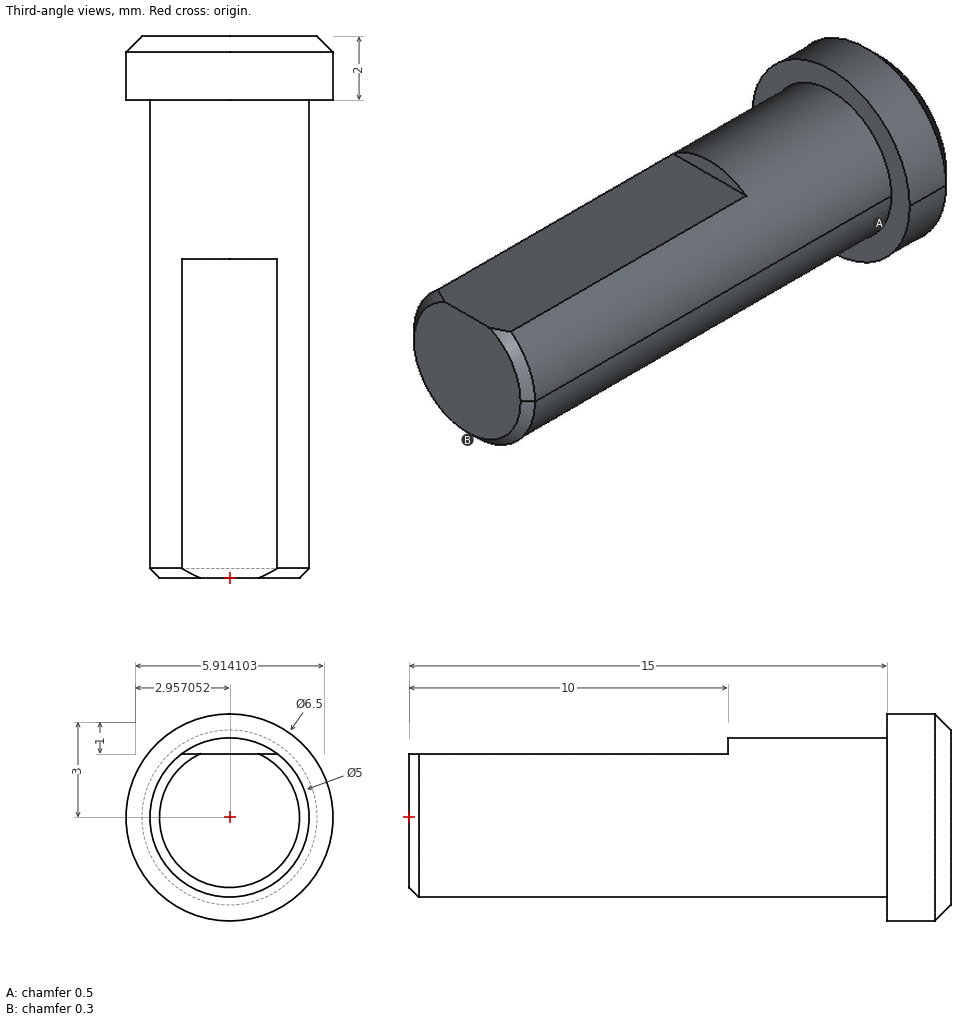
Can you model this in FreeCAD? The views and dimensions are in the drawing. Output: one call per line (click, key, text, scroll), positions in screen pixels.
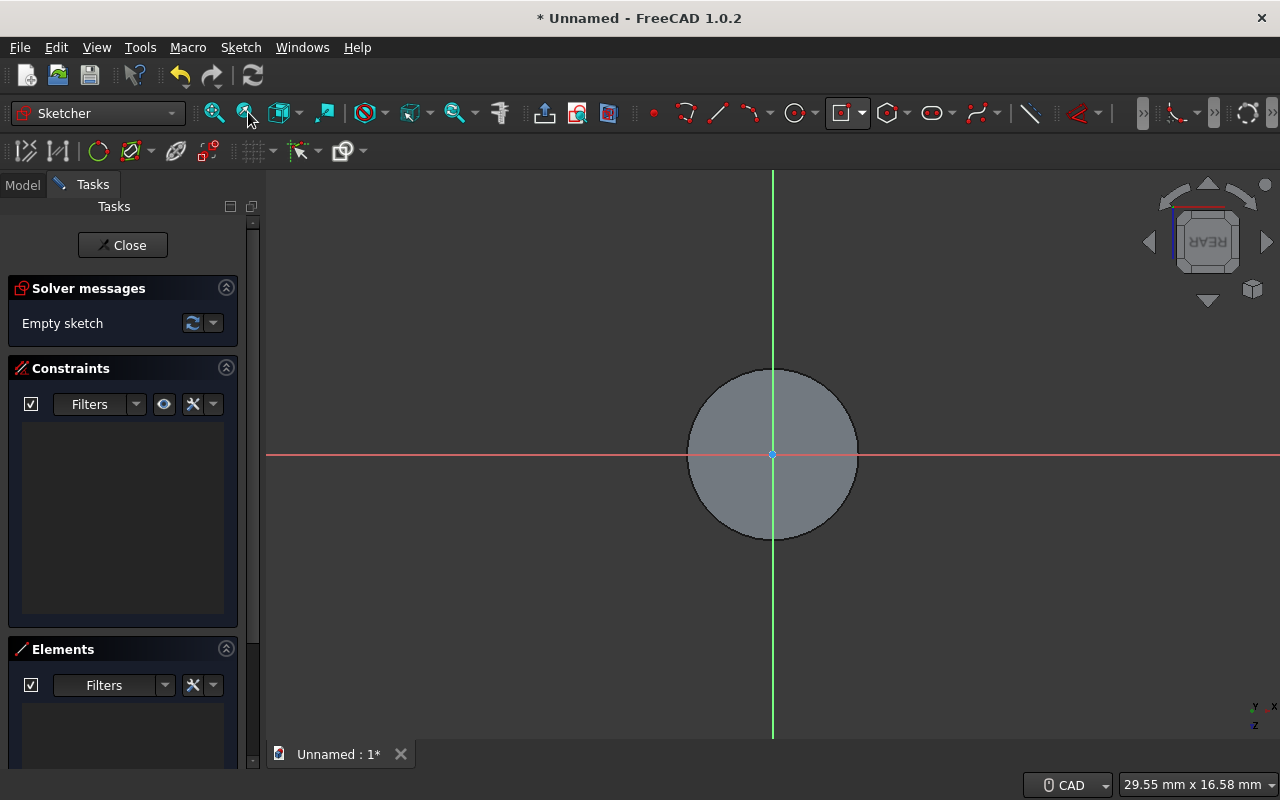
scroll(912, 454, up, 2)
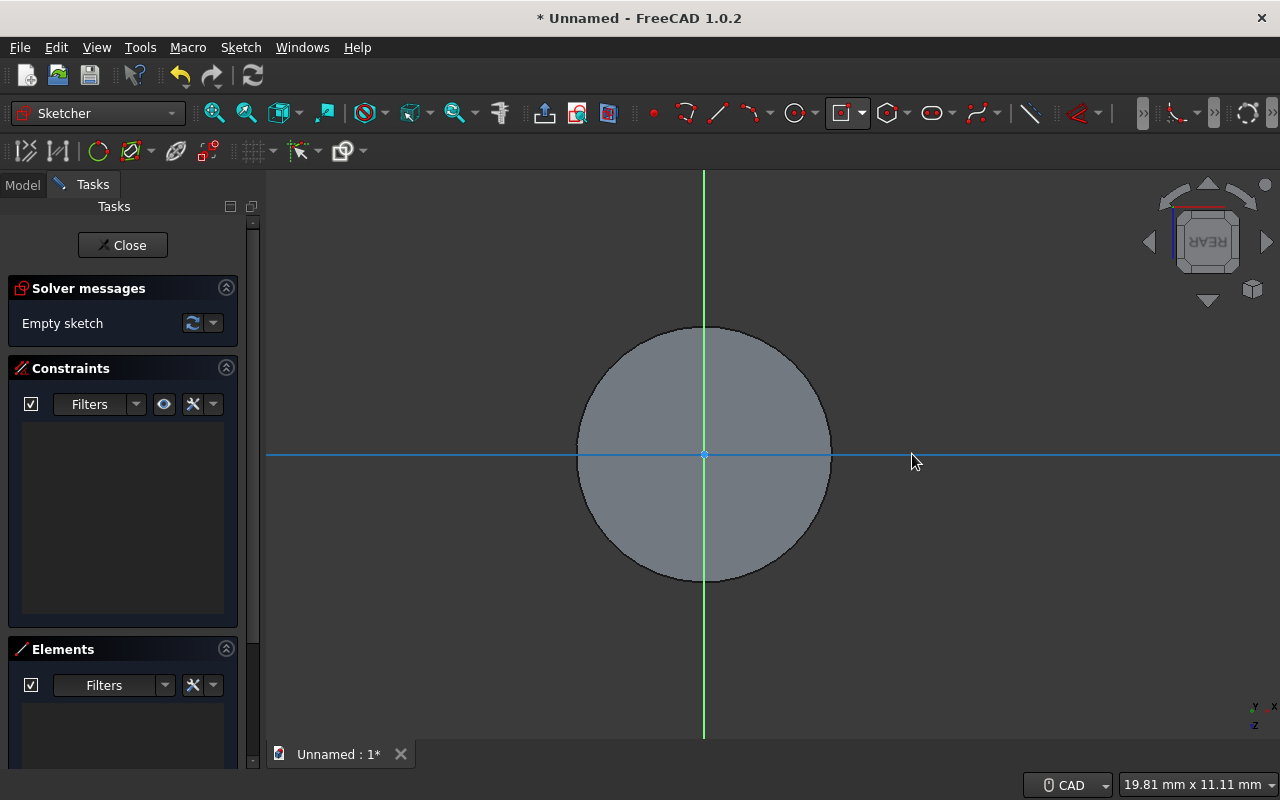
click(796, 114)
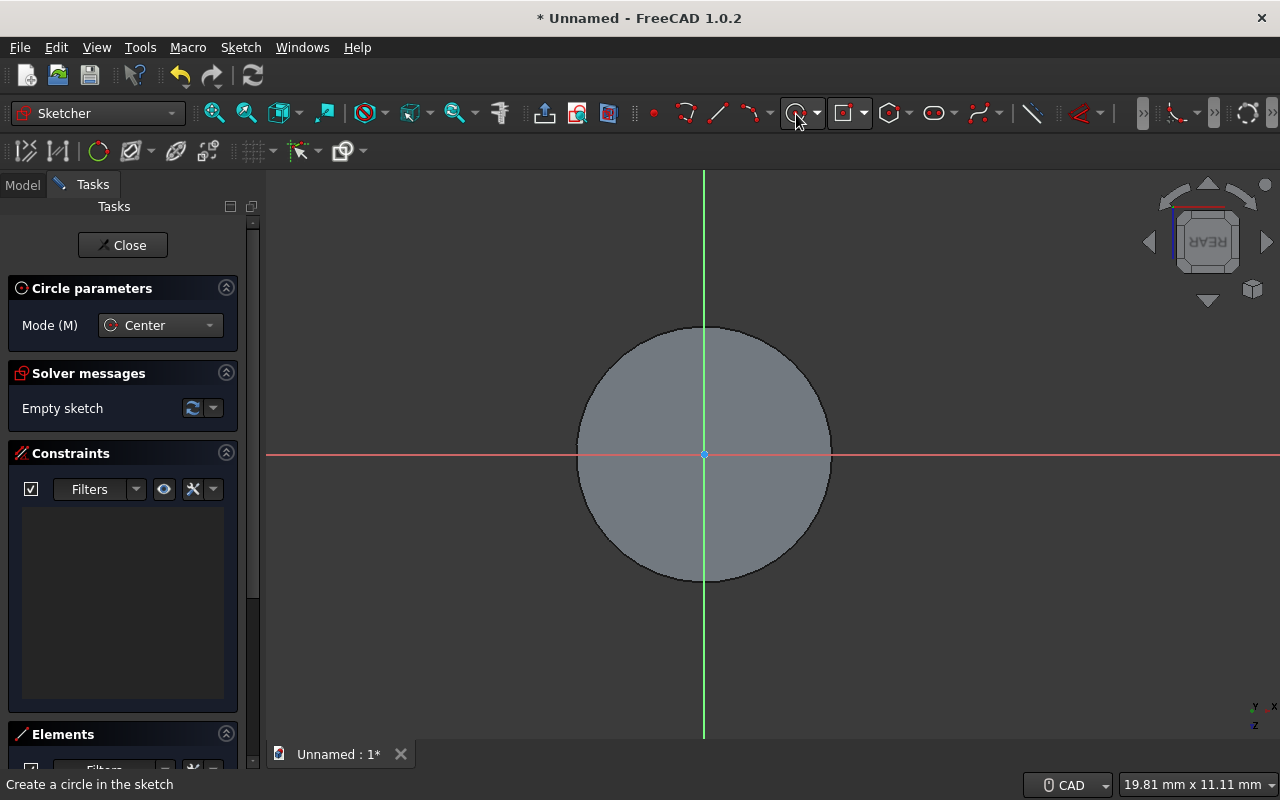
click(704, 454)
click(822, 337)
key(Escape)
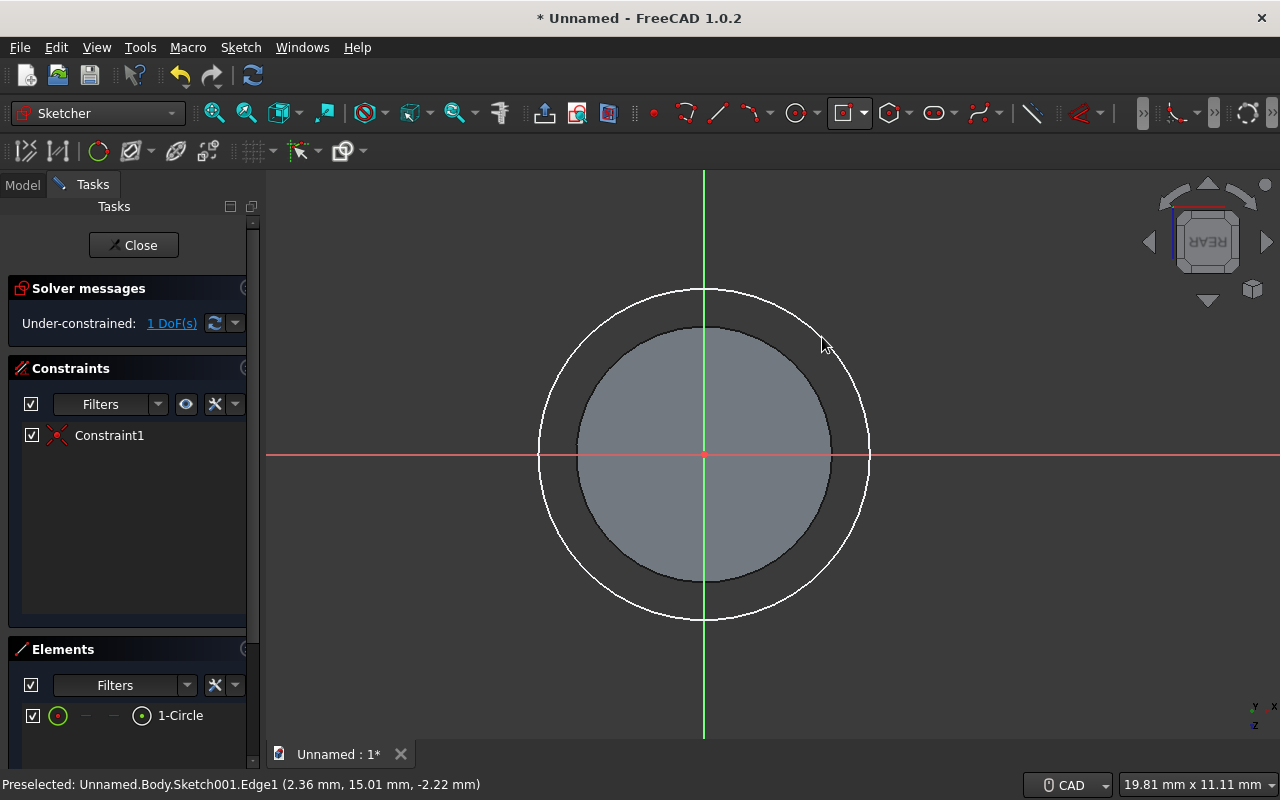
click(1080, 114)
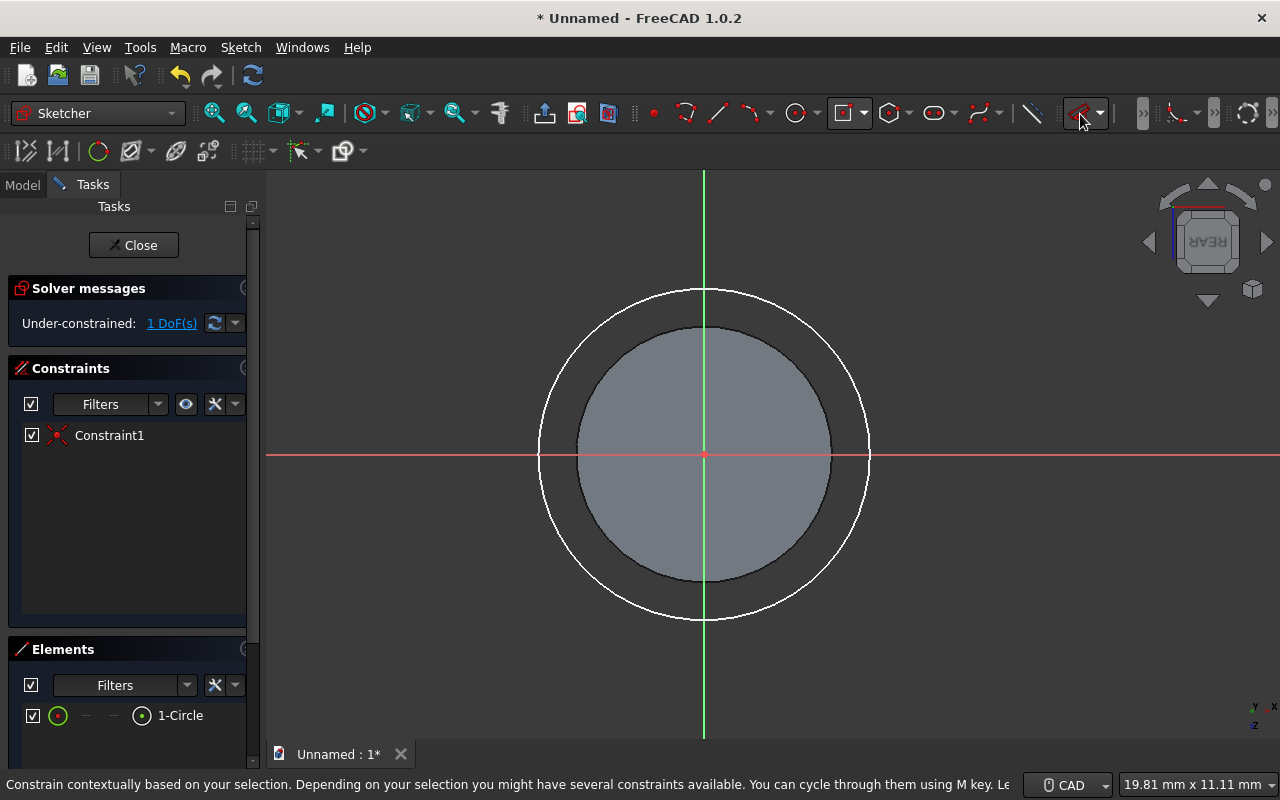
click(821, 337)
click(844, 314)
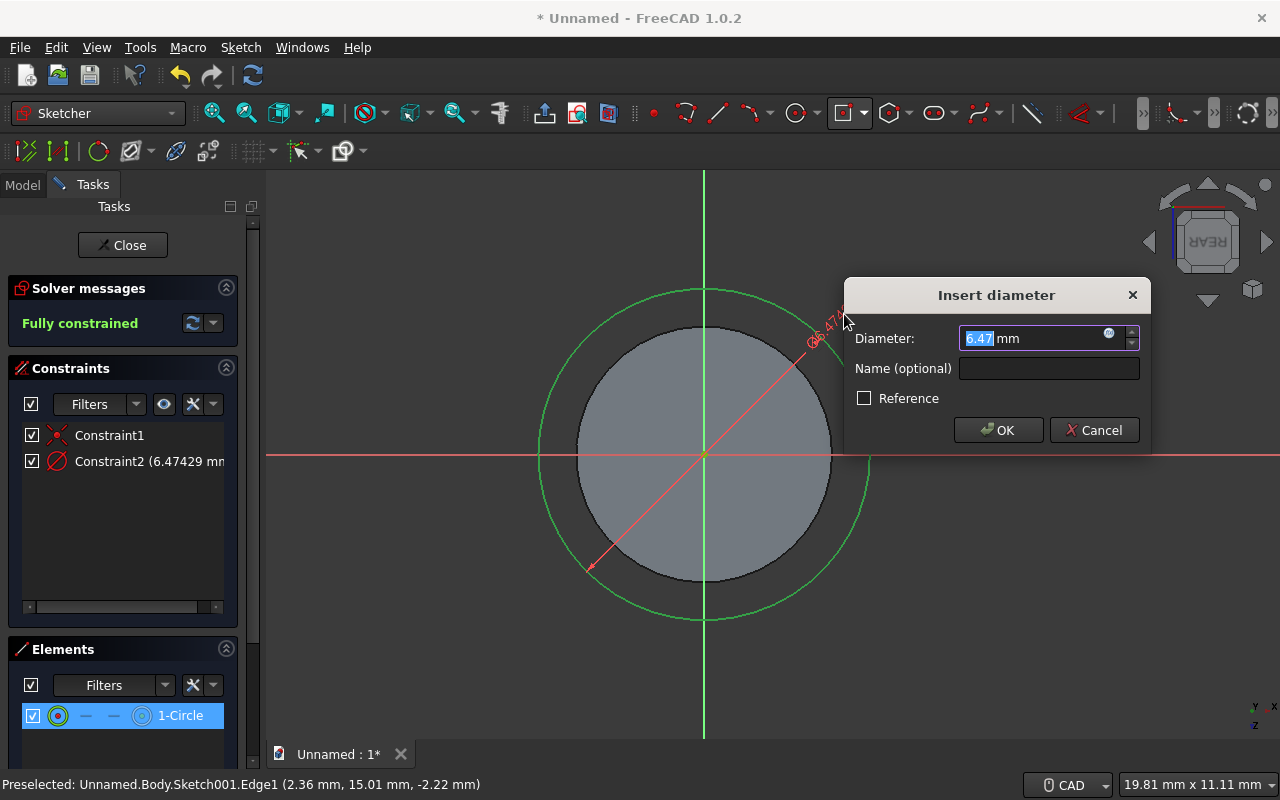
text(6.5)
key(Return)
key(Escape)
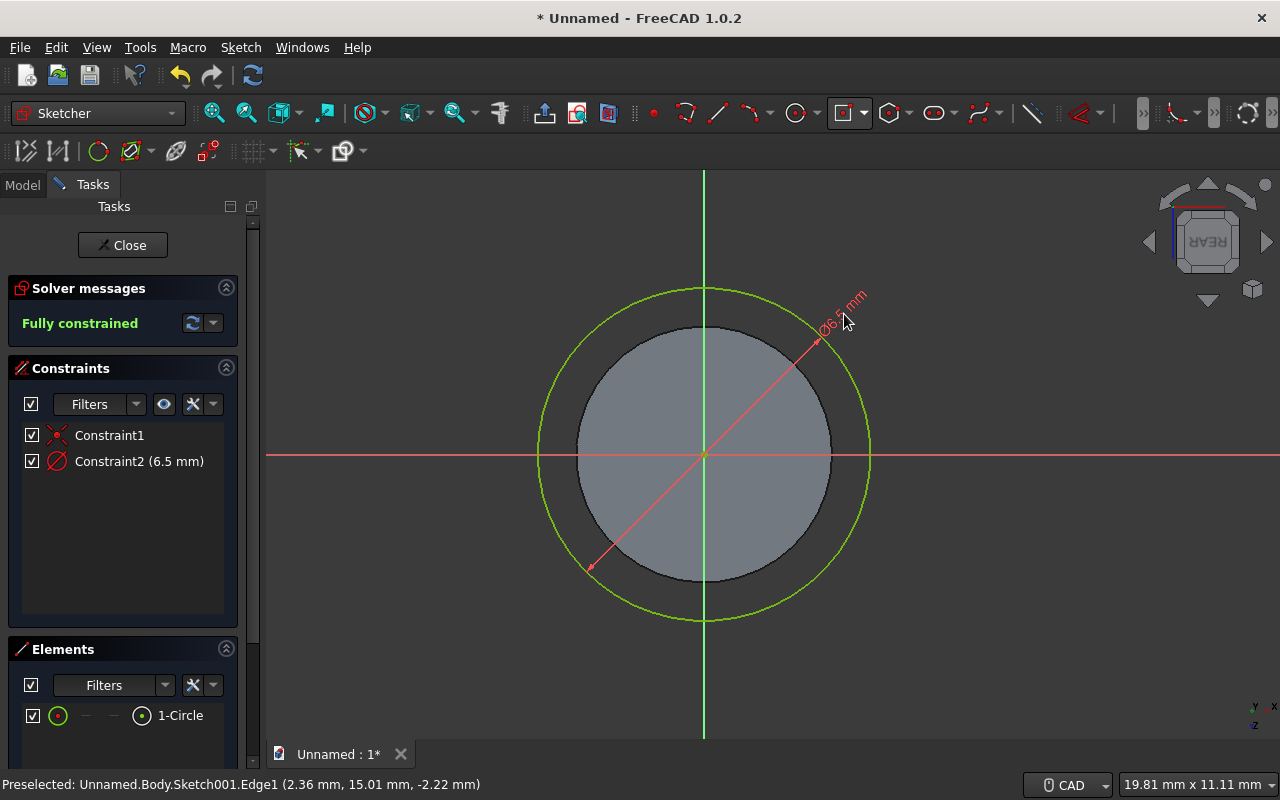
click(123, 245)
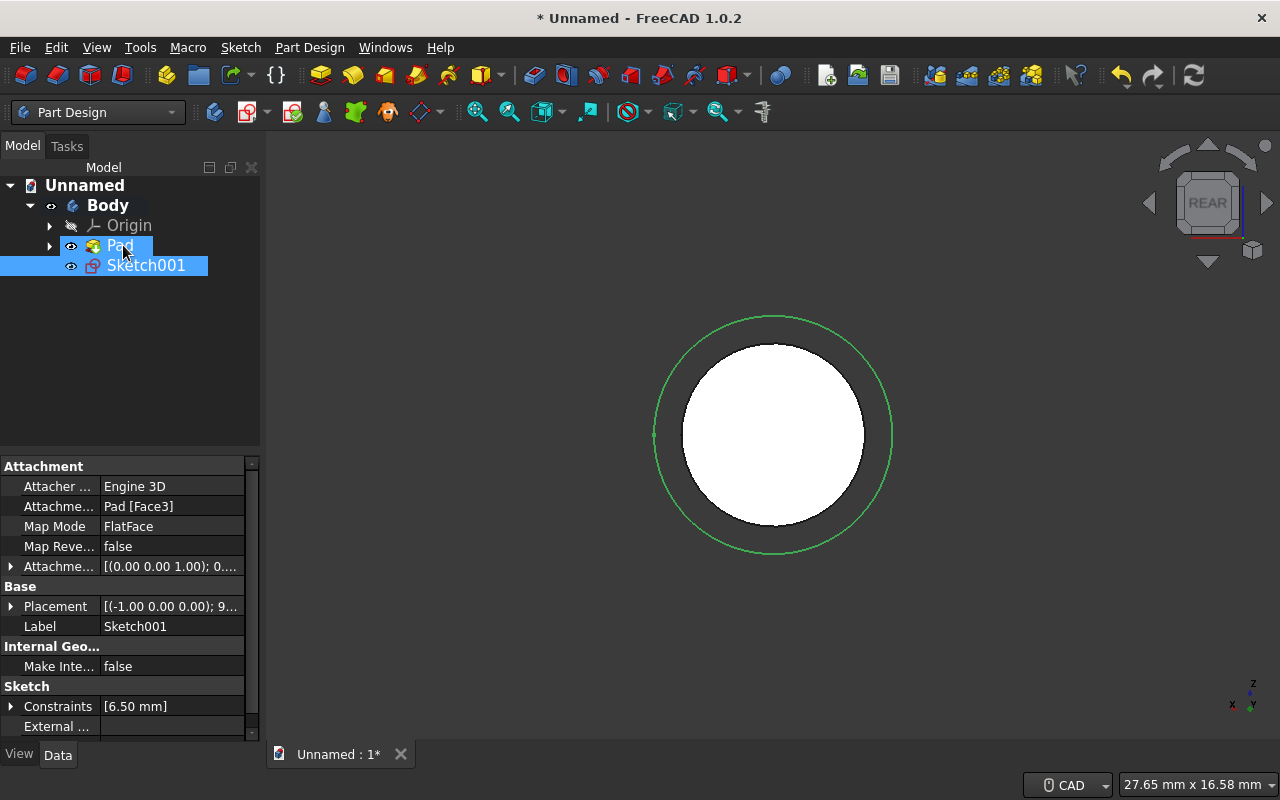
click(322, 76)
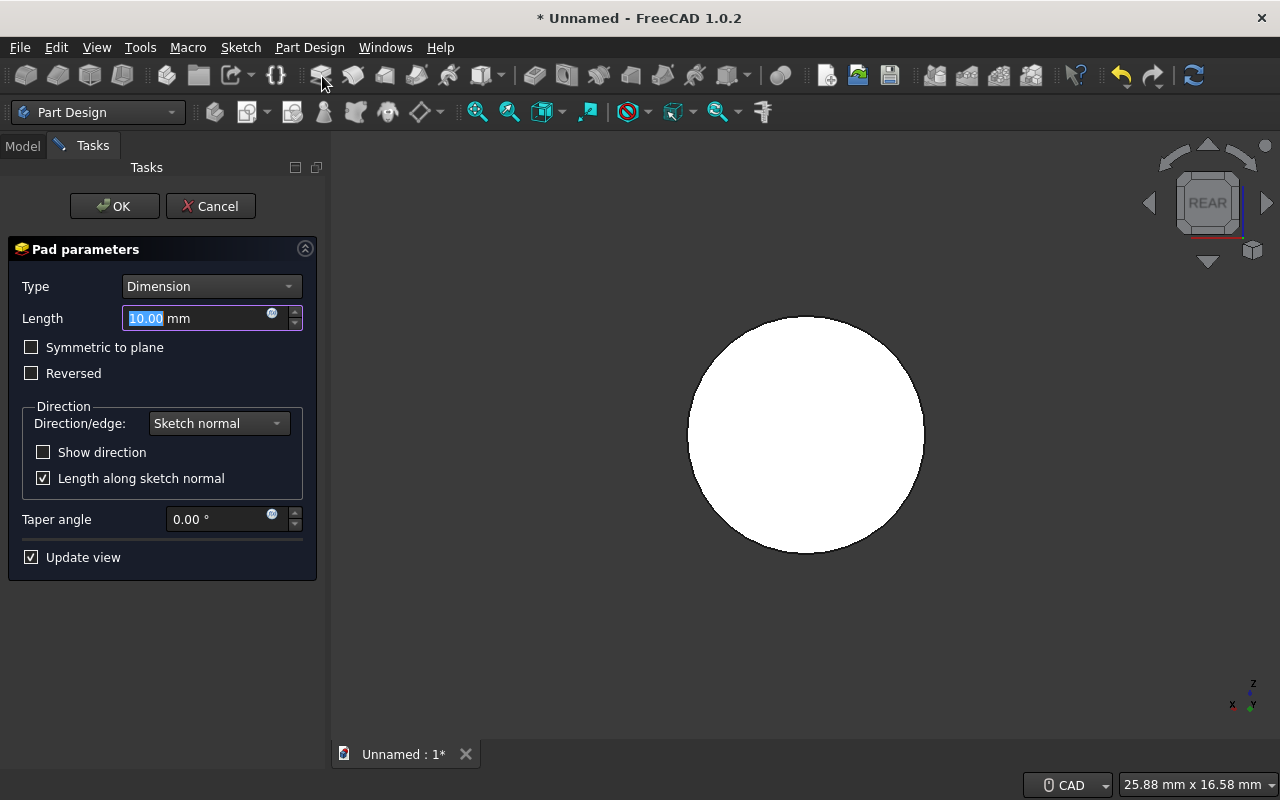
text(2)
key(Tab)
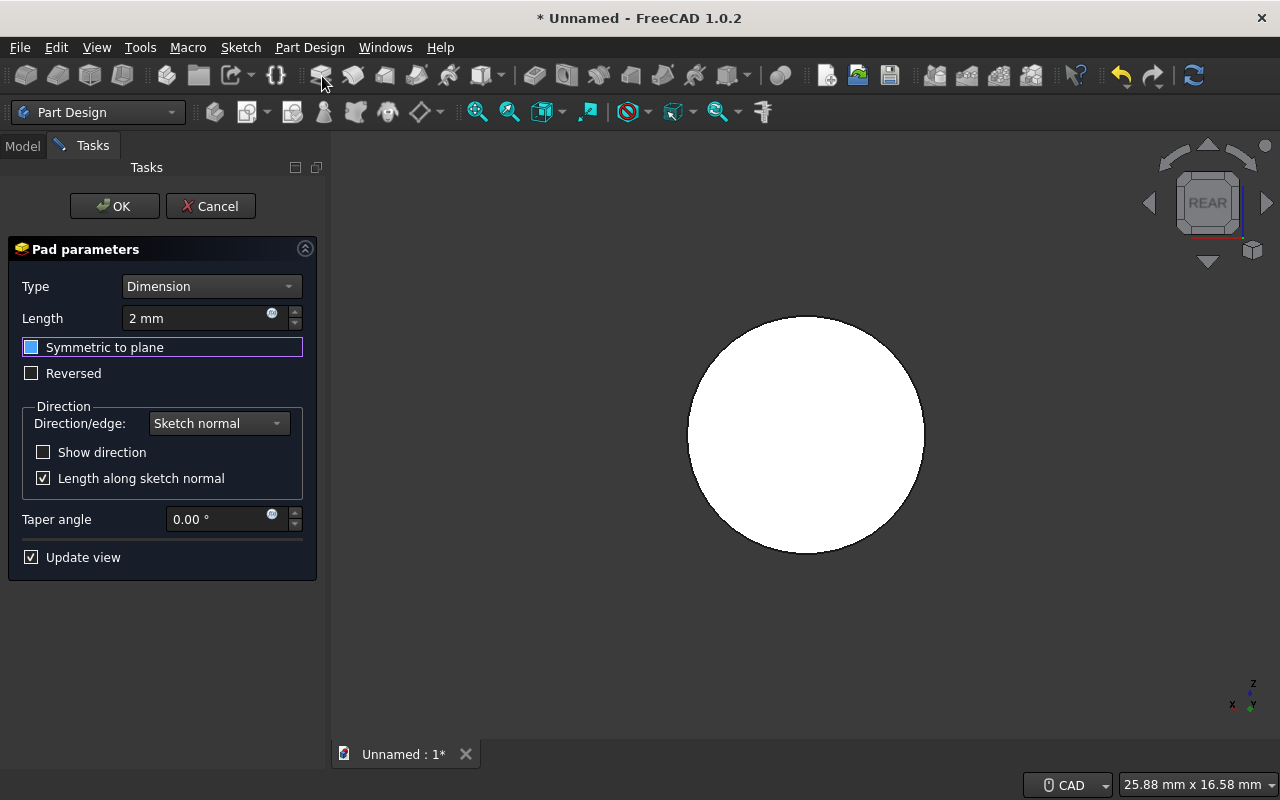
click(115, 206)